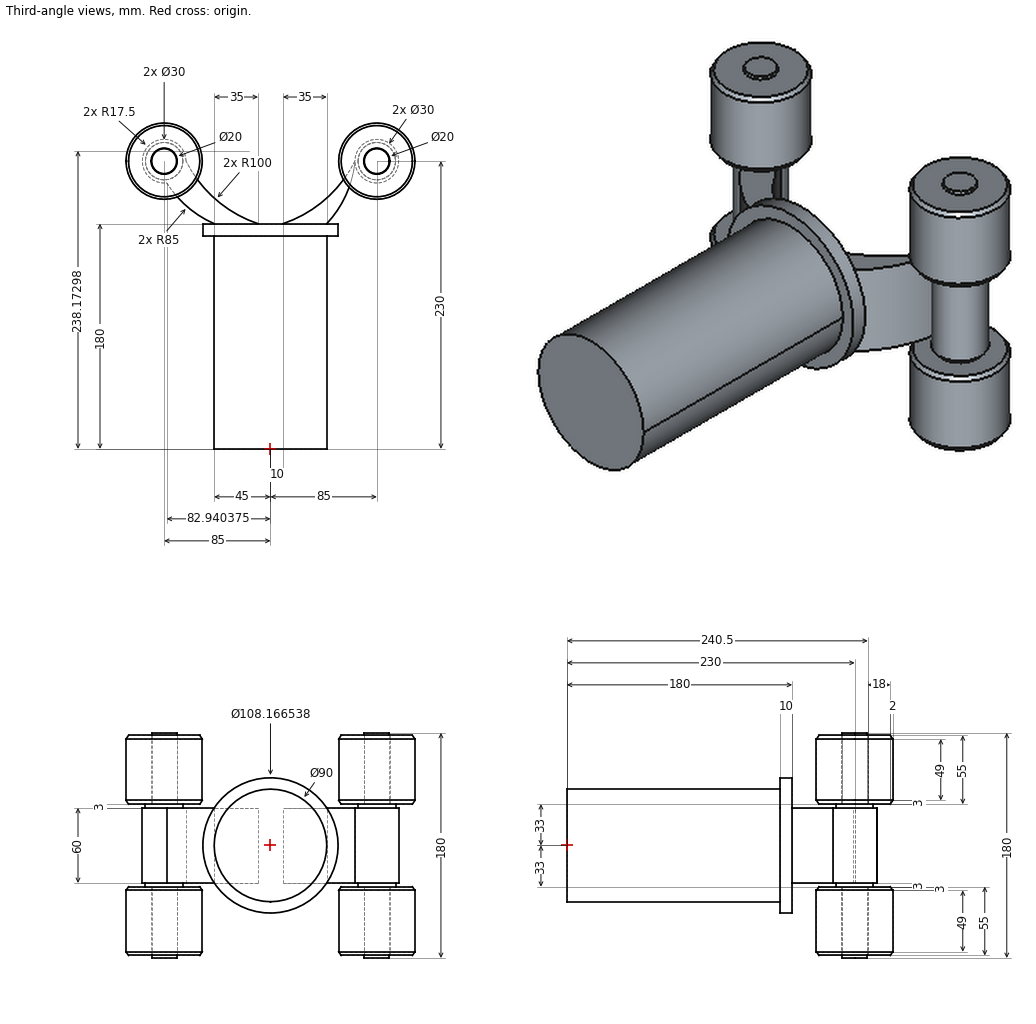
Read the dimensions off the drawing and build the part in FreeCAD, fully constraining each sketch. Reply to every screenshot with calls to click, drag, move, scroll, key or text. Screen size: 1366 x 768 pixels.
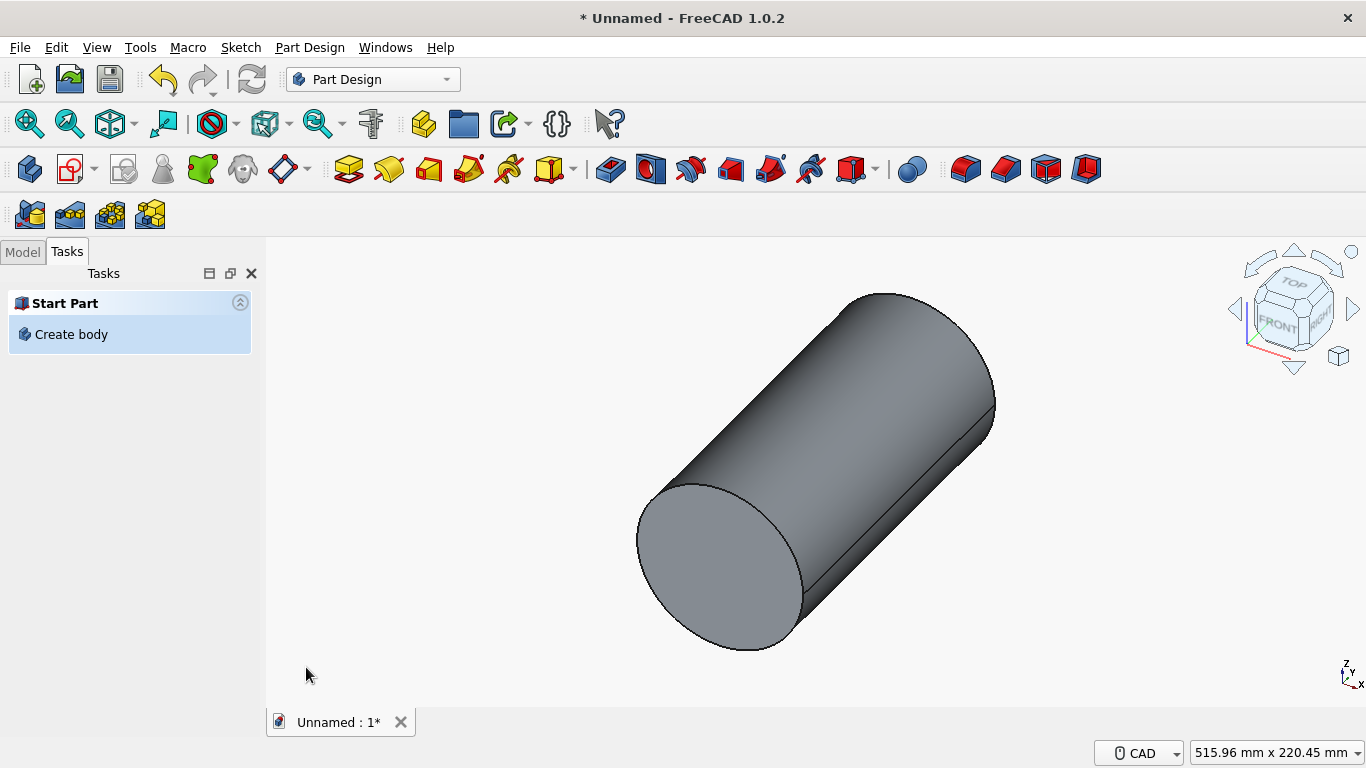
click(70, 170)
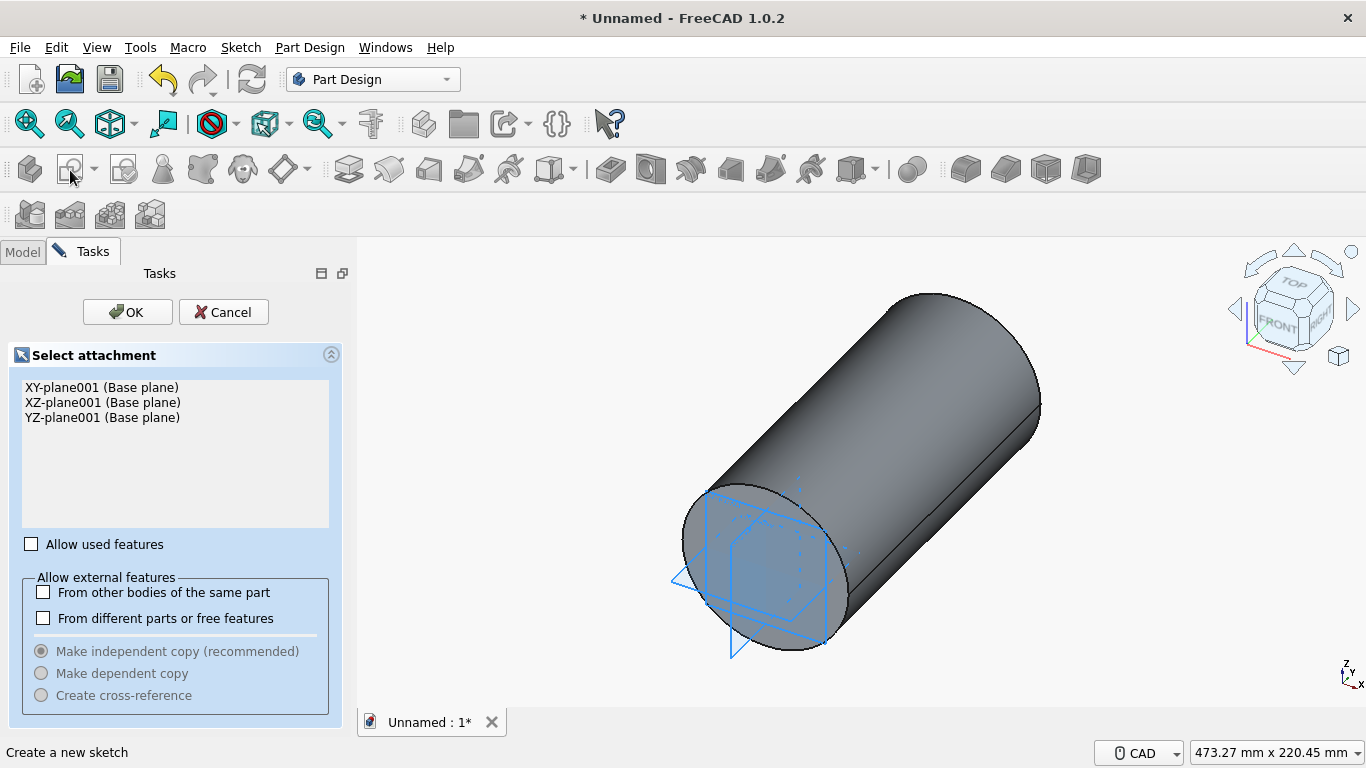
click(82, 388)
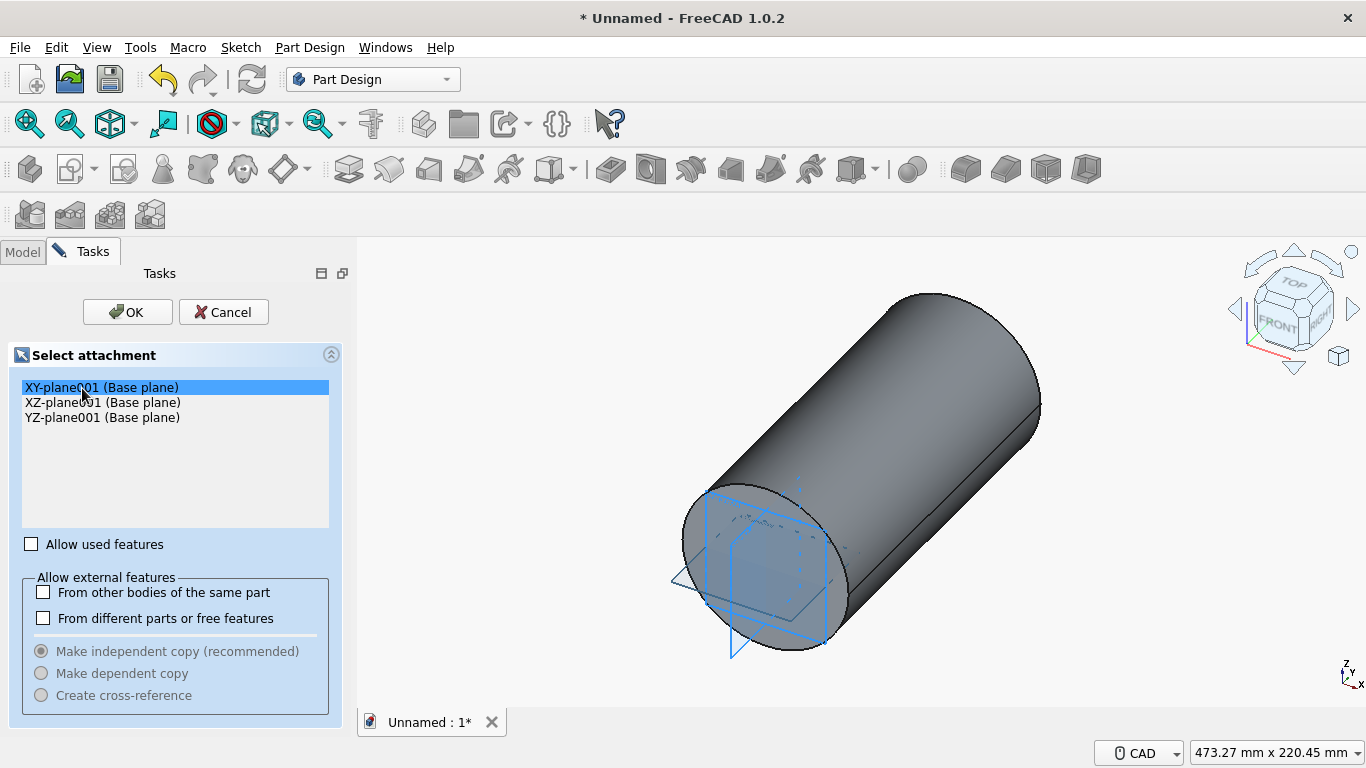
click(128, 312)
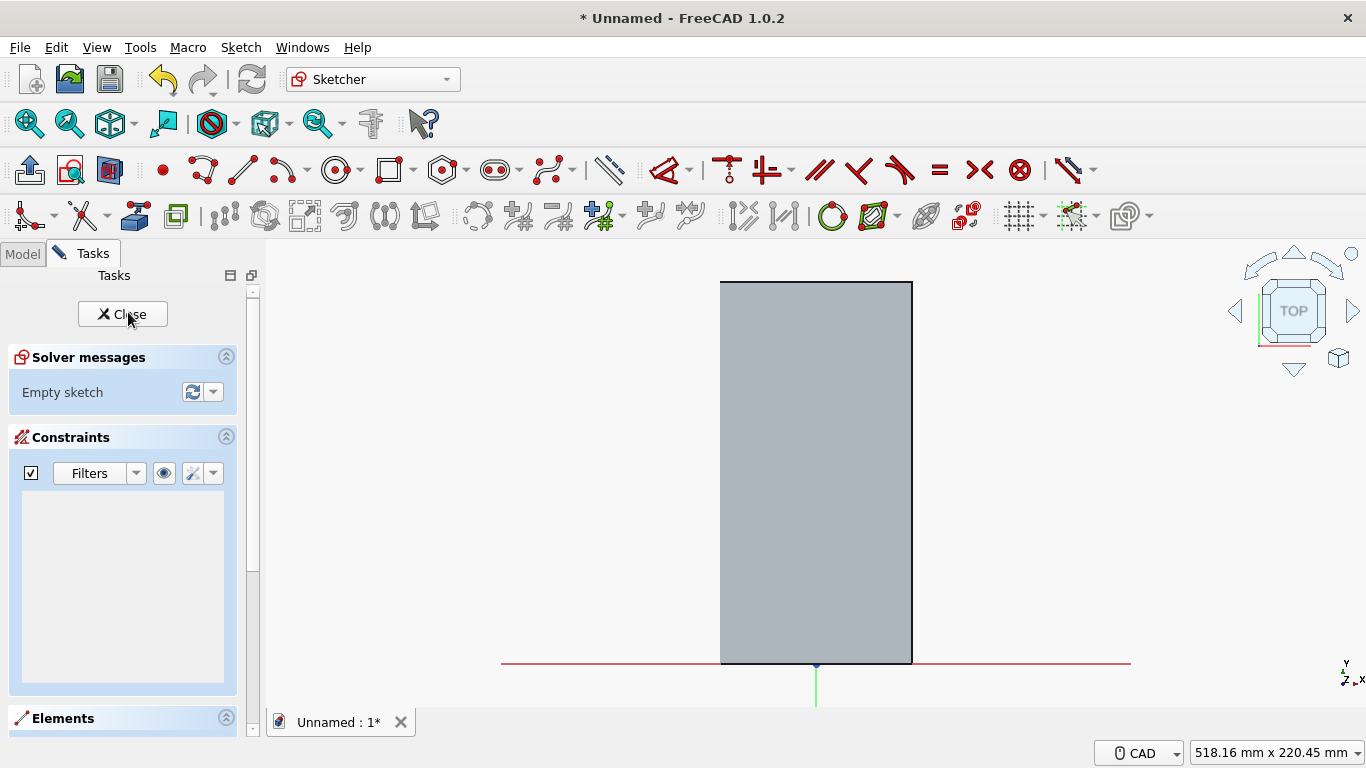
scroll(748, 473, down, 5)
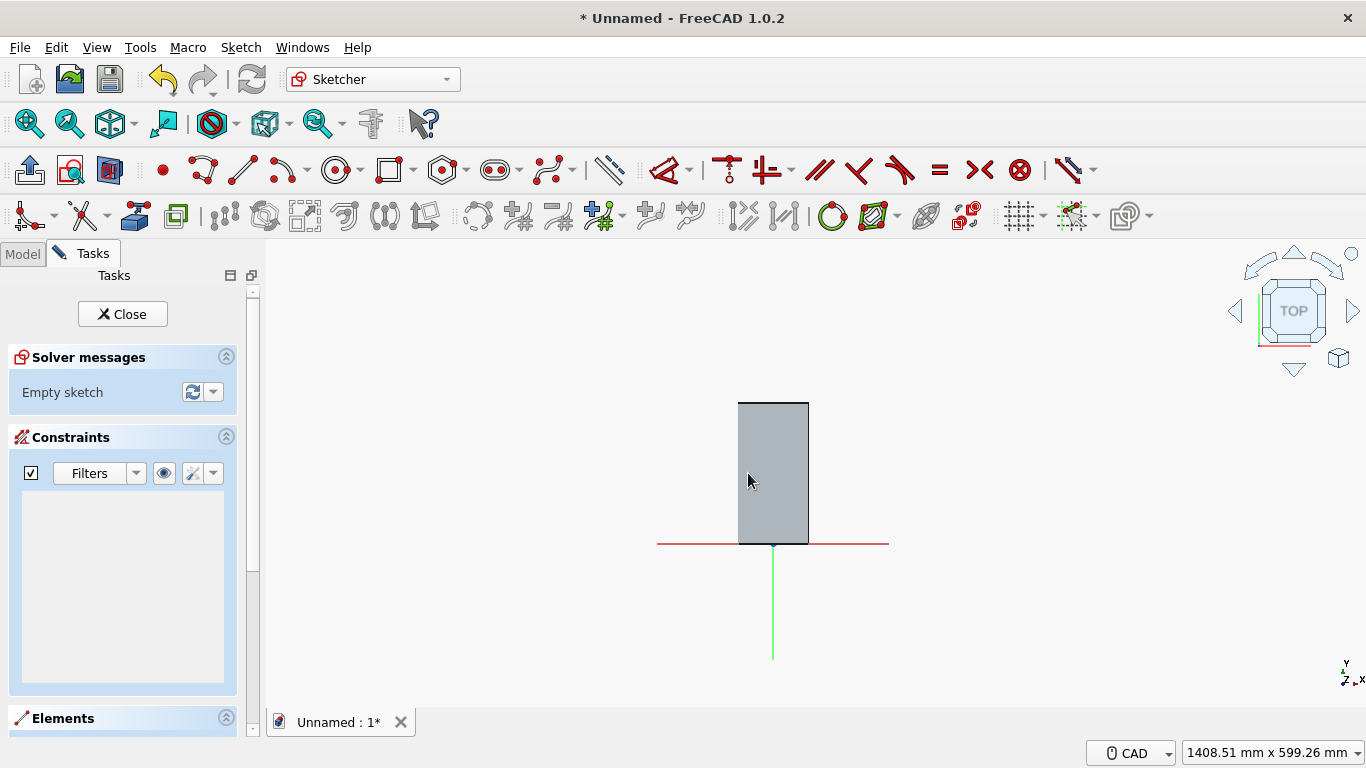
scroll(845, 358, up, 15)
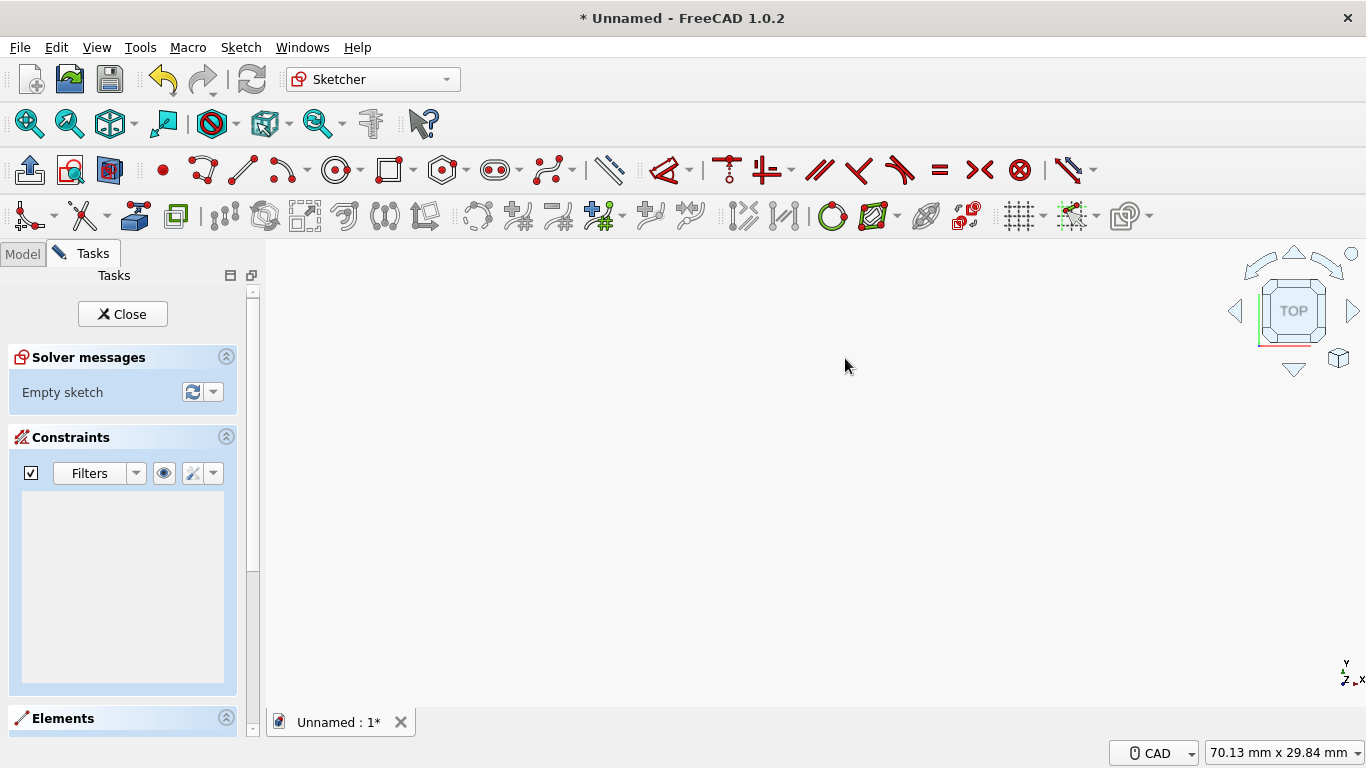
click(336, 170)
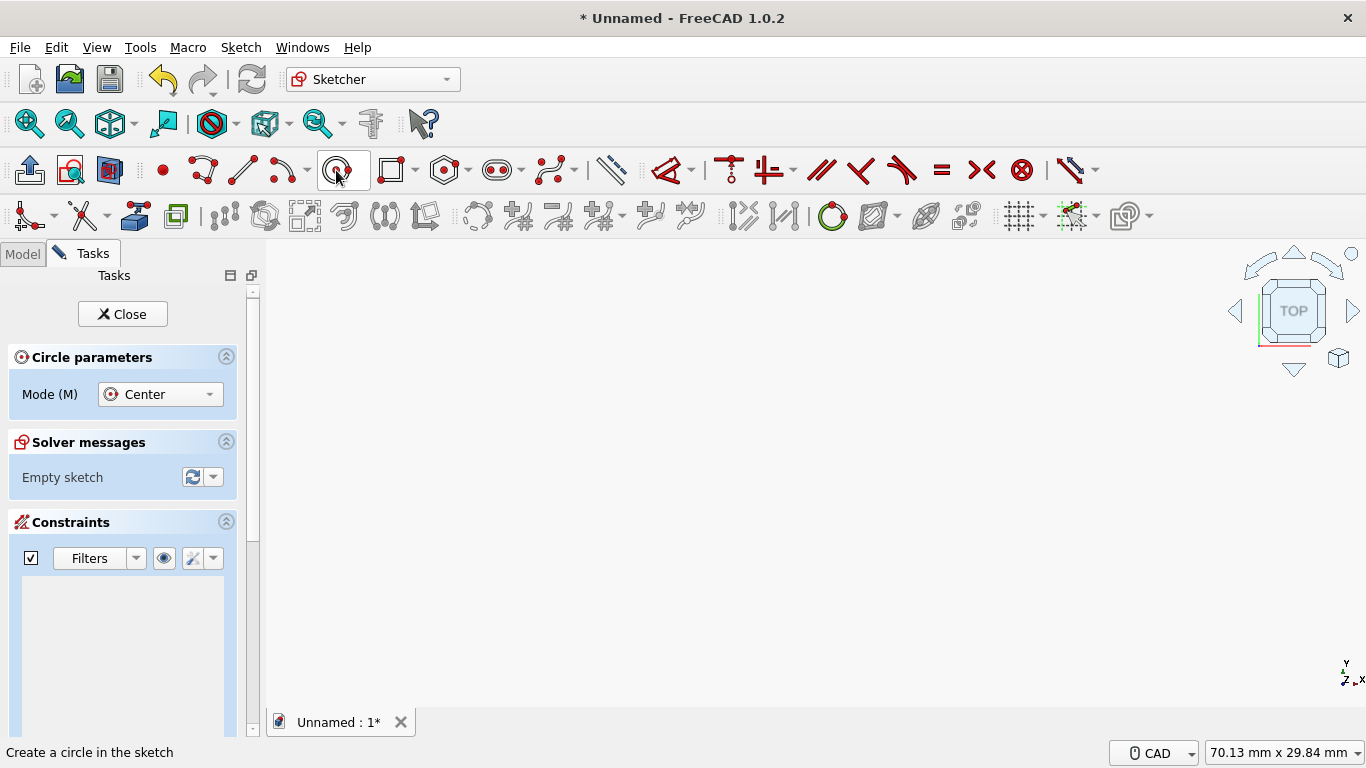
click(728, 473)
click(839, 362)
key(Escape)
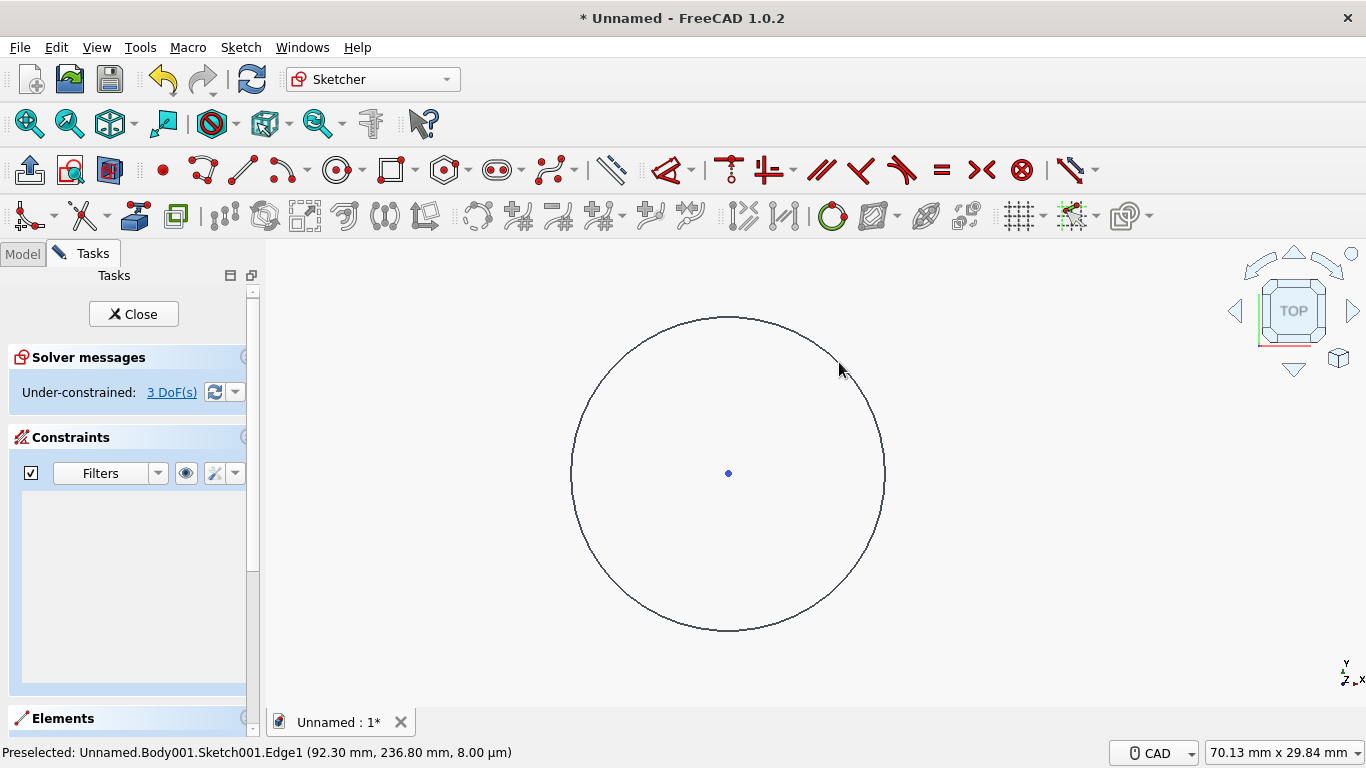
click(666, 170)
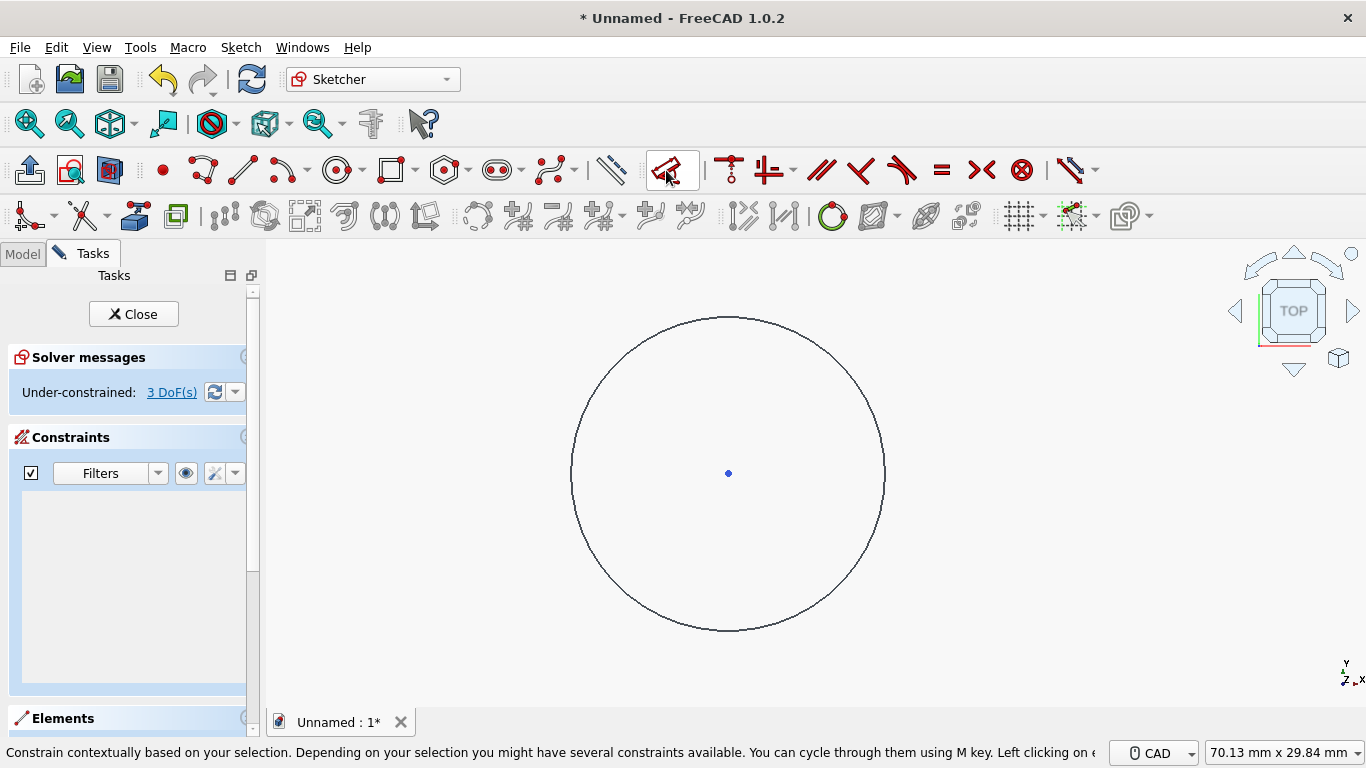
click(839, 363)
click(862, 340)